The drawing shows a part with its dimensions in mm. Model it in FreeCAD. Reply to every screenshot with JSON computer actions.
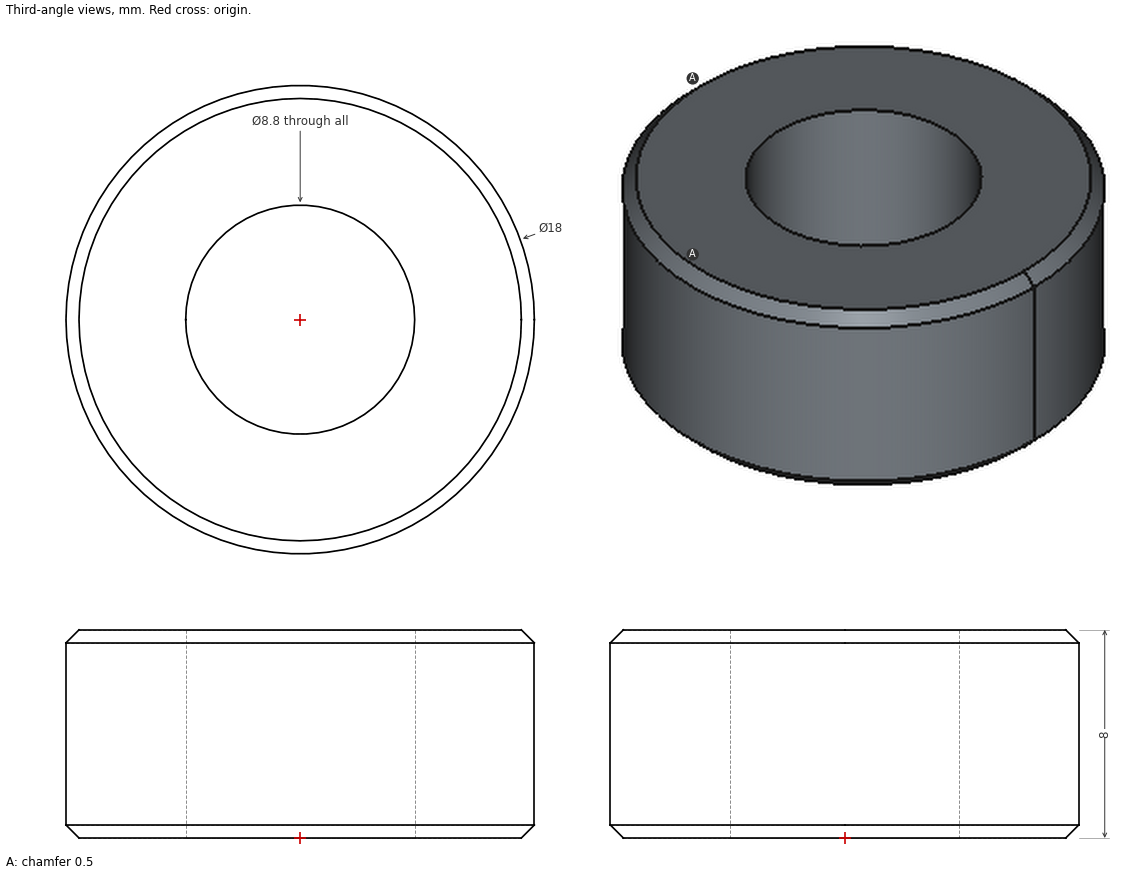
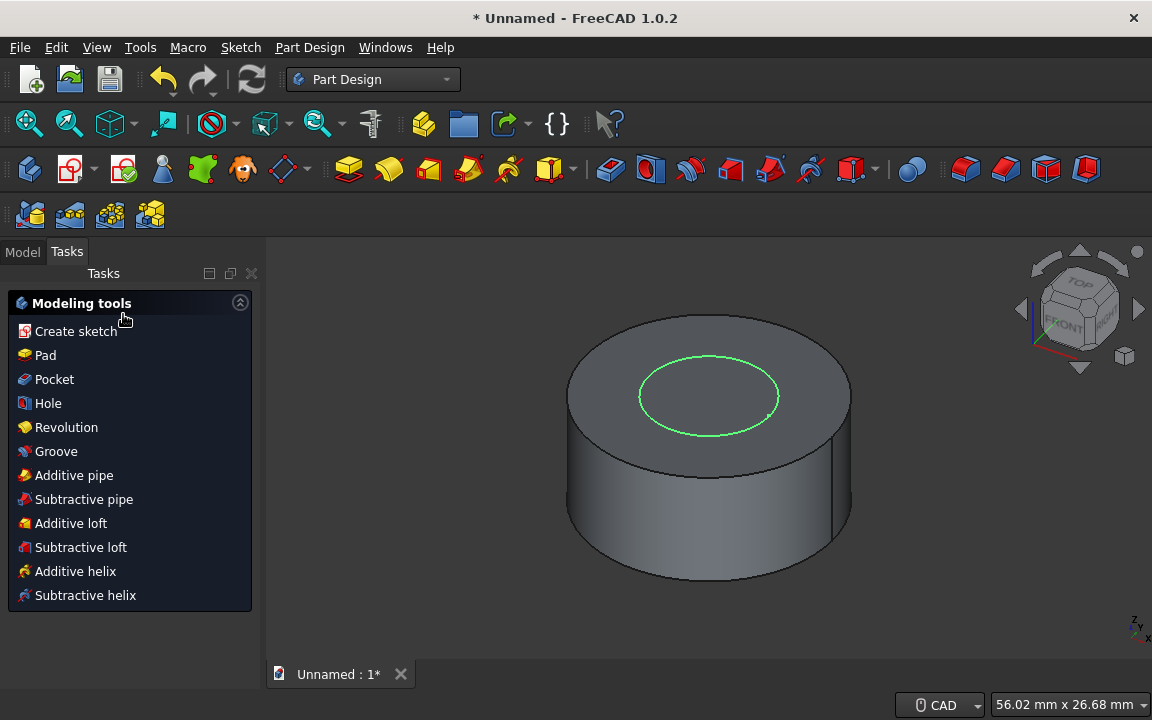
{"action": "left_click", "coordinate": [652, 170]}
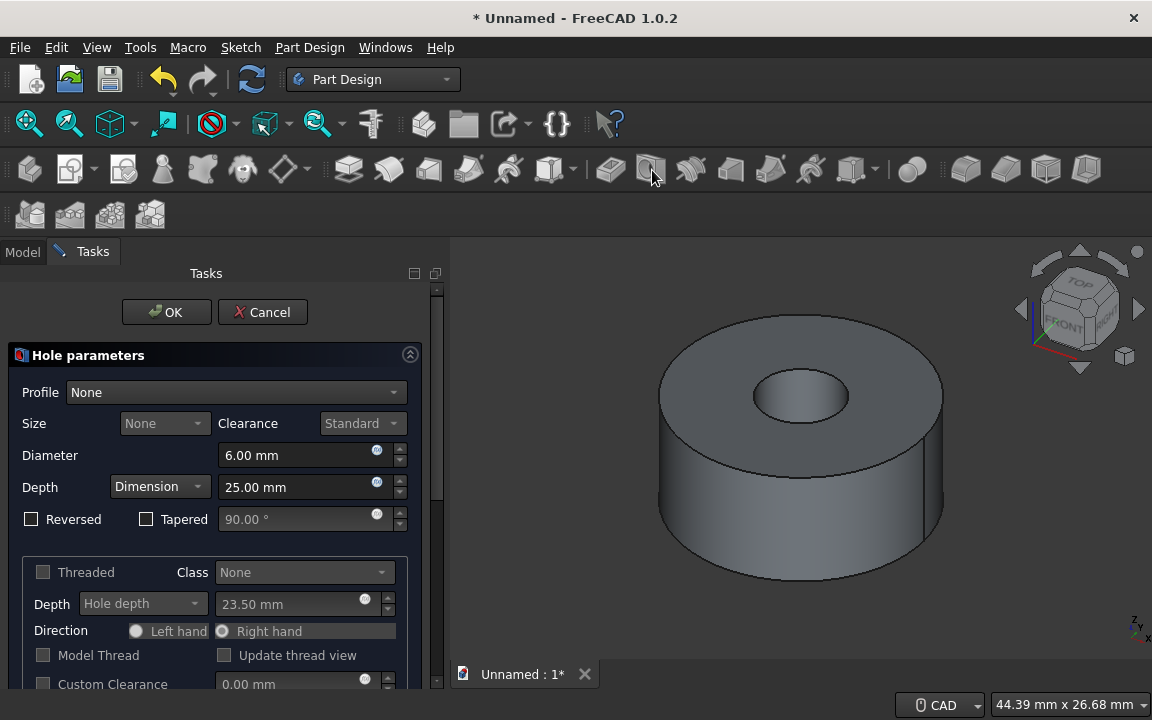
{"action": "triple_click", "coordinate": [305, 455]}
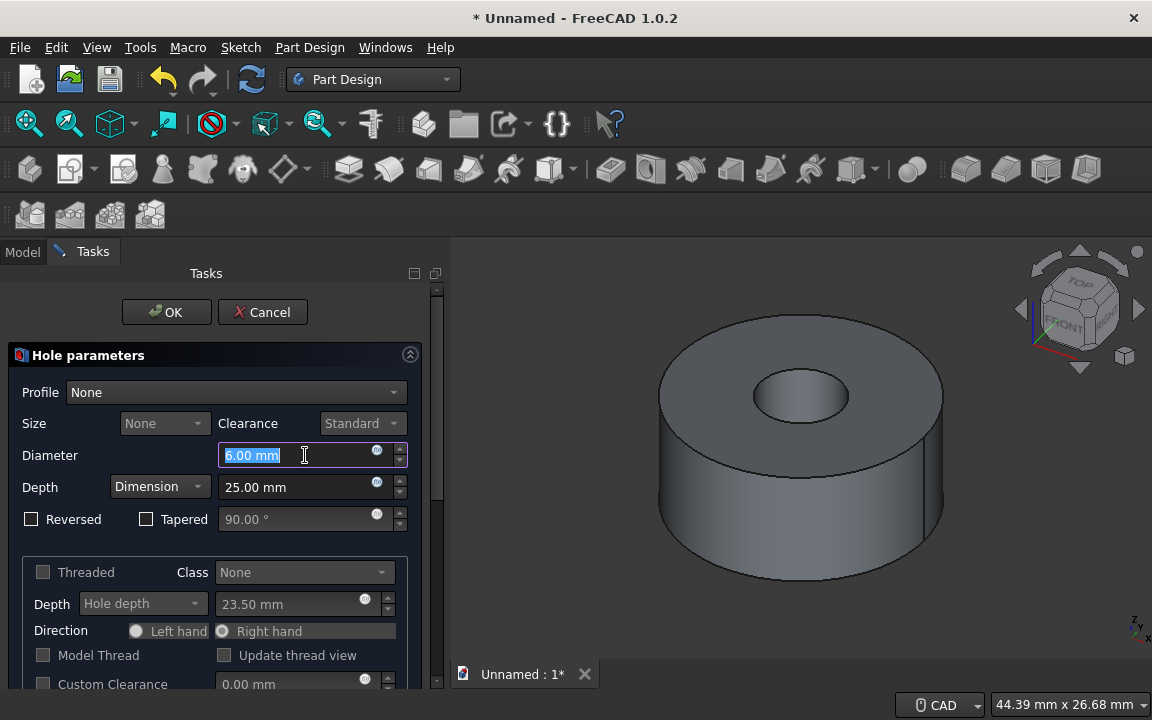
{"action": "type", "text": "8.8"}
{"action": "key", "text": "Tab"}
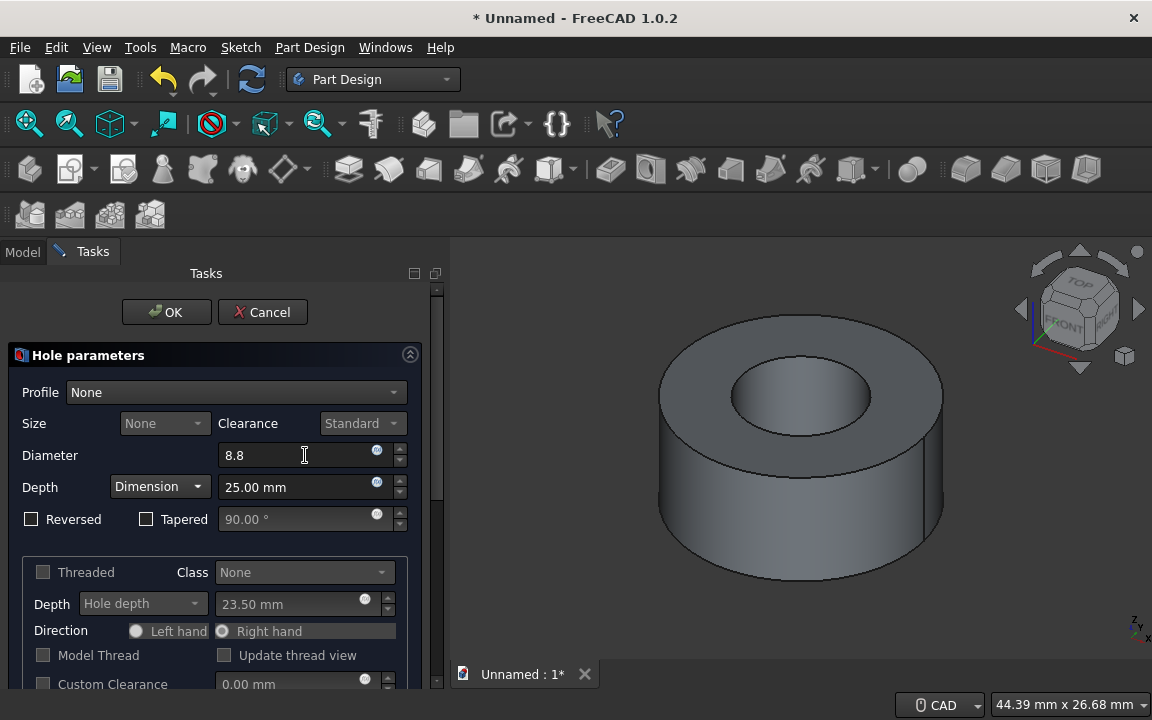
{"action": "left_click", "coordinate": [161, 486]}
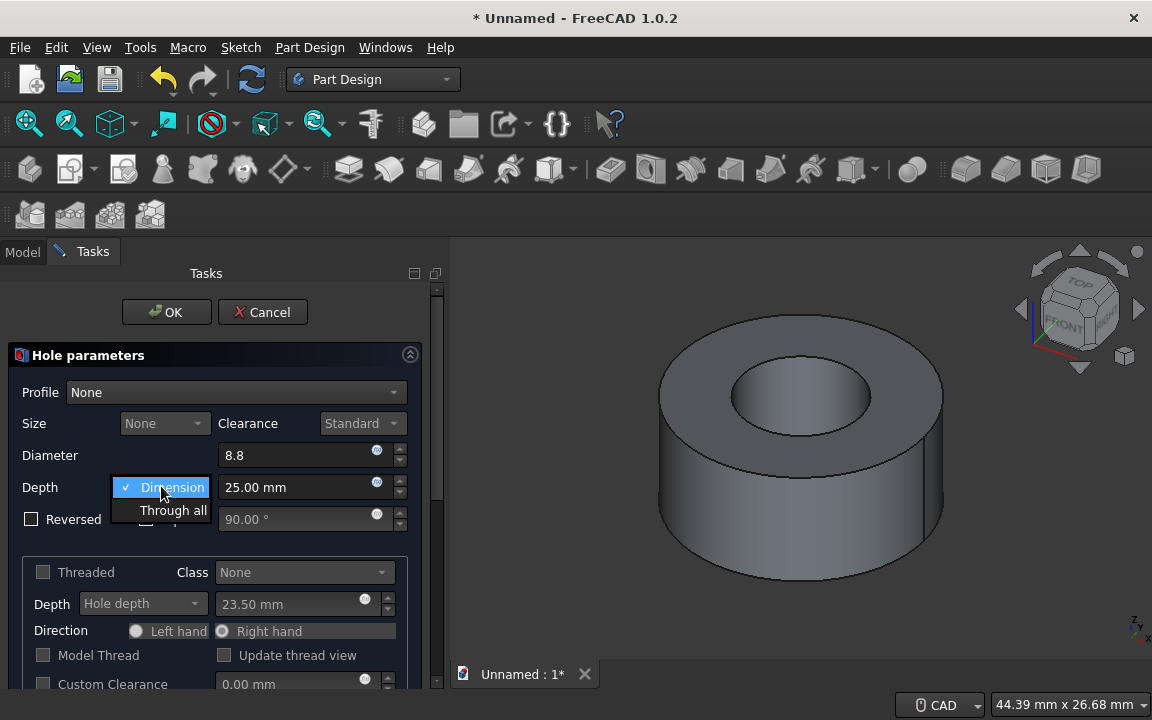
{"action": "left_click", "coordinate": [160, 510]}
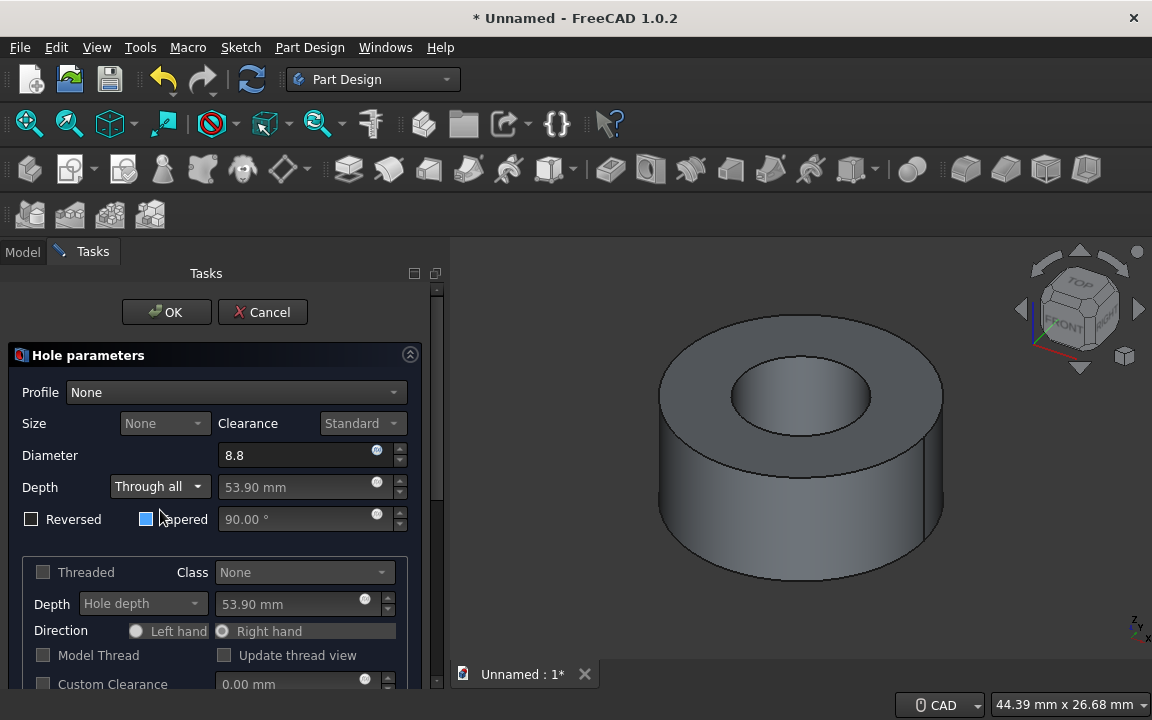
{"action": "left_click", "coordinate": [167, 312]}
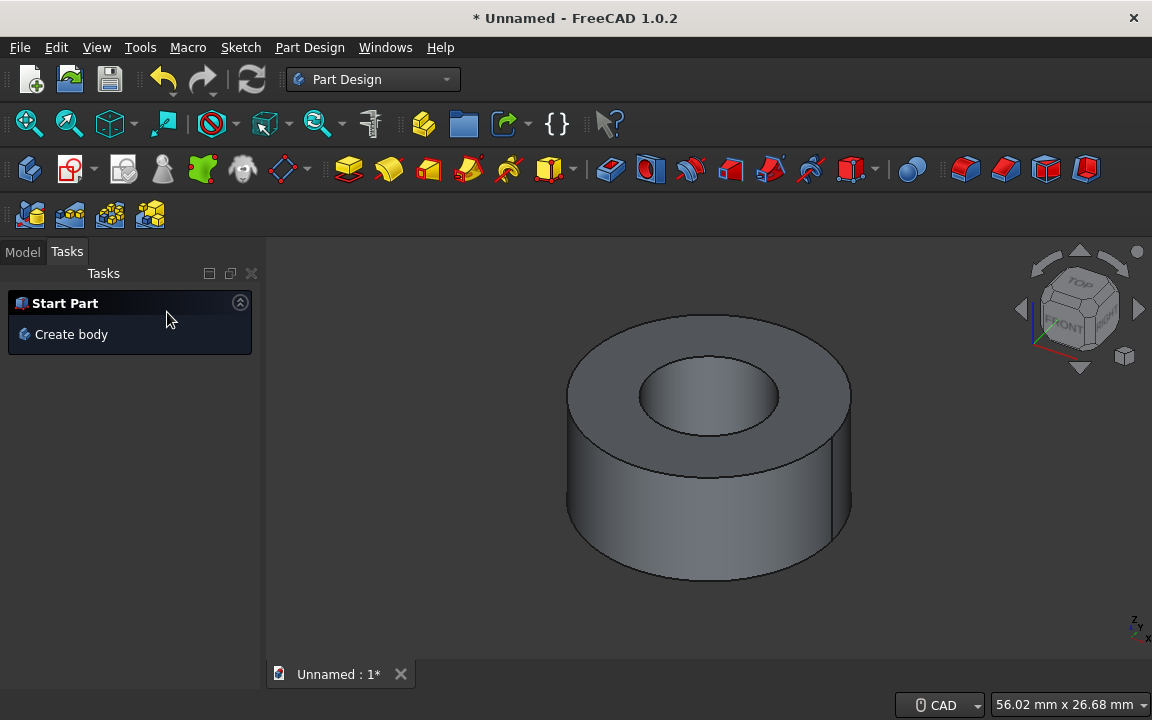
{"action": "left_click", "coordinate": [679, 579]}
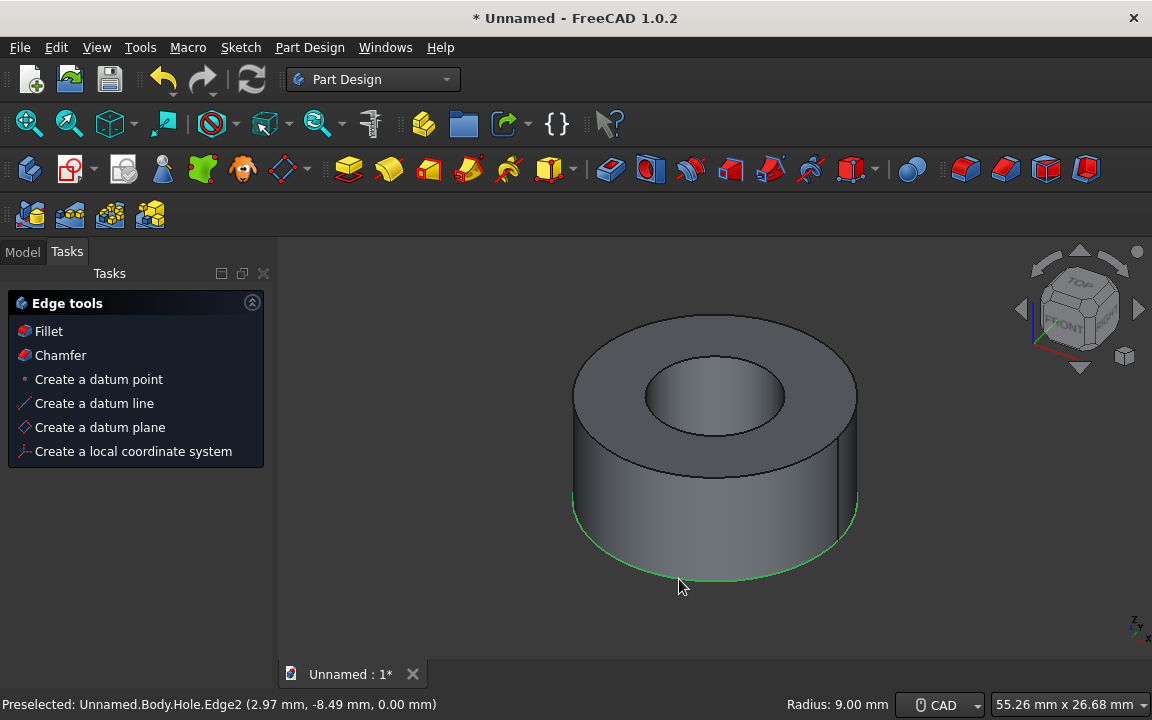
{"action": "left_click", "coordinate": [573, 404], "text": "ctrl"}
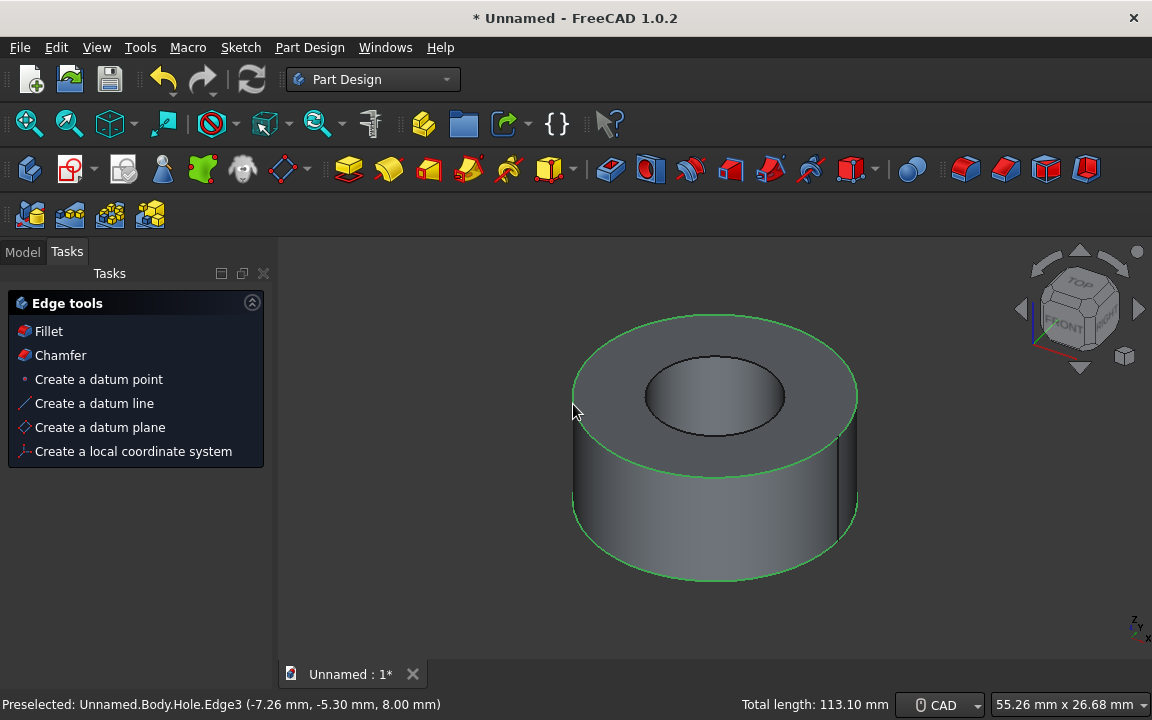
{"action": "left_click", "coordinate": [1006, 170]}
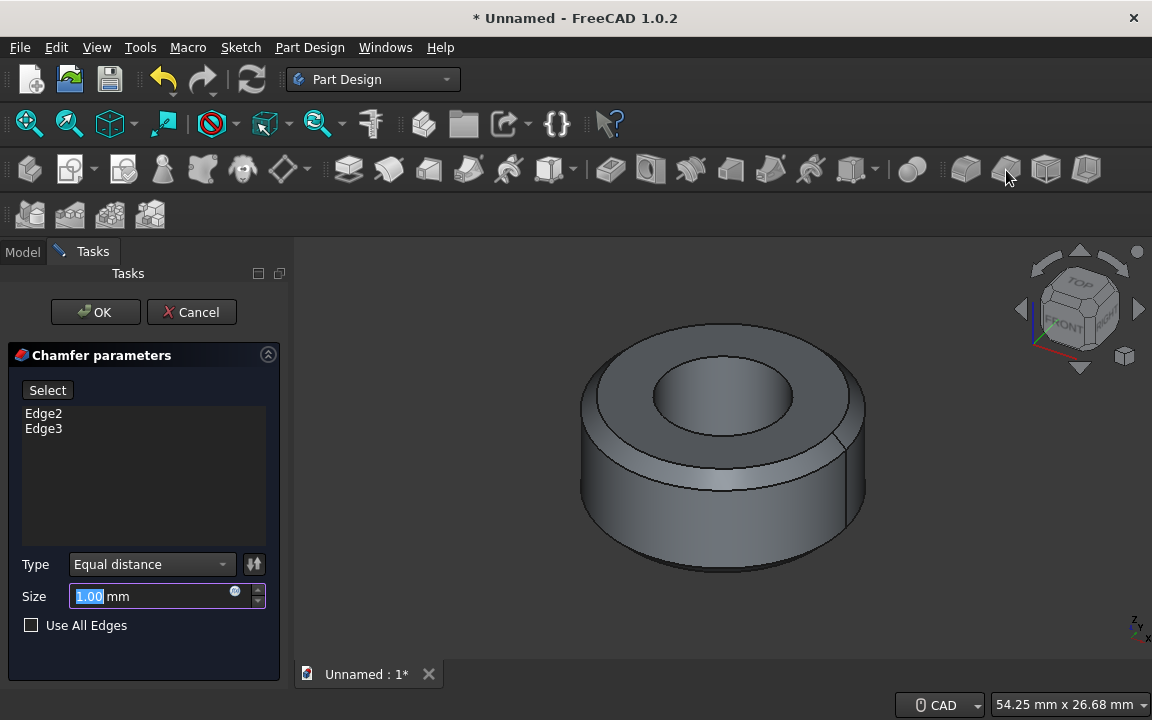
{"action": "type", "text": "0.5"}
{"action": "key", "text": "Tab"}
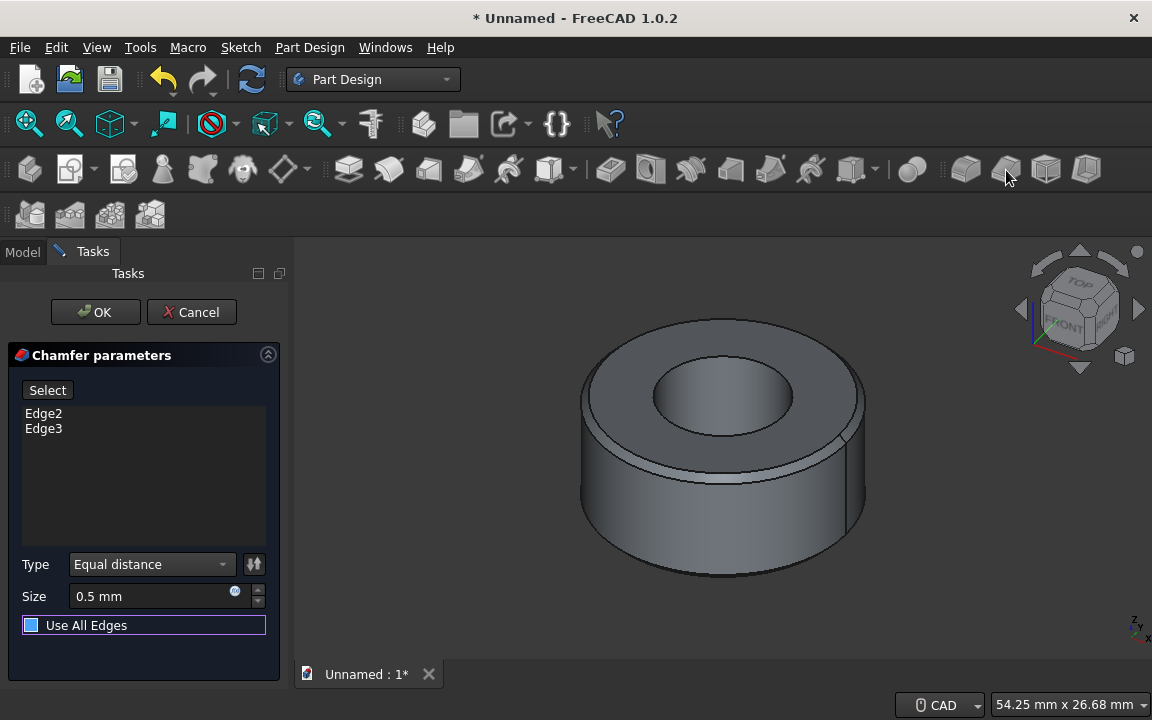
{"action": "left_click", "coordinate": [96, 312]}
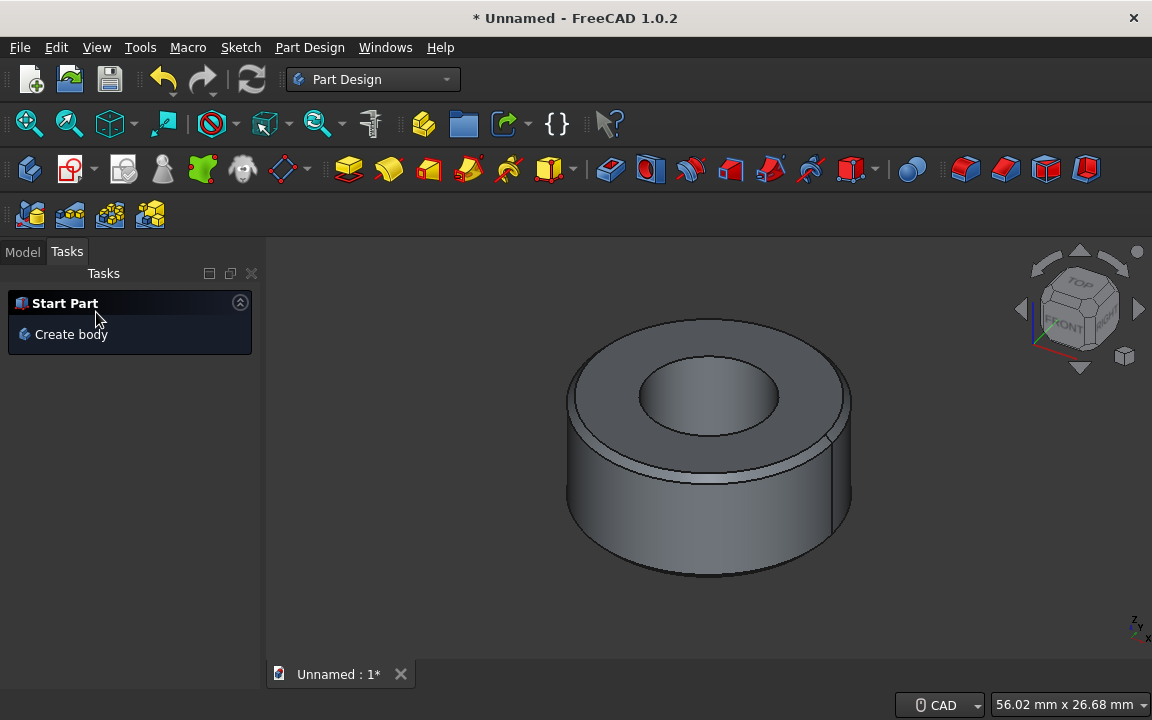
{"action": "key", "text": "0"}